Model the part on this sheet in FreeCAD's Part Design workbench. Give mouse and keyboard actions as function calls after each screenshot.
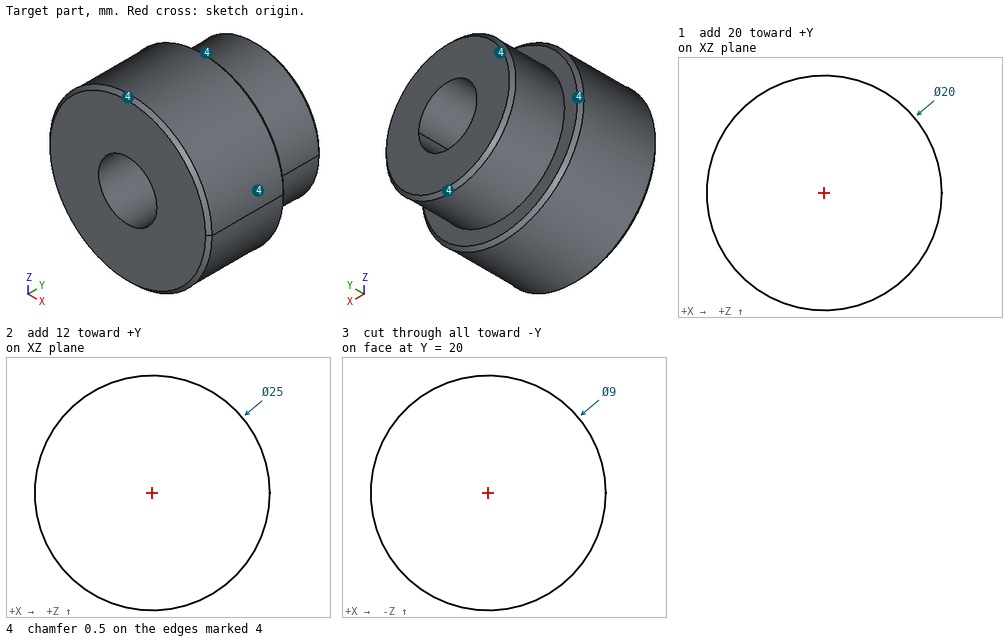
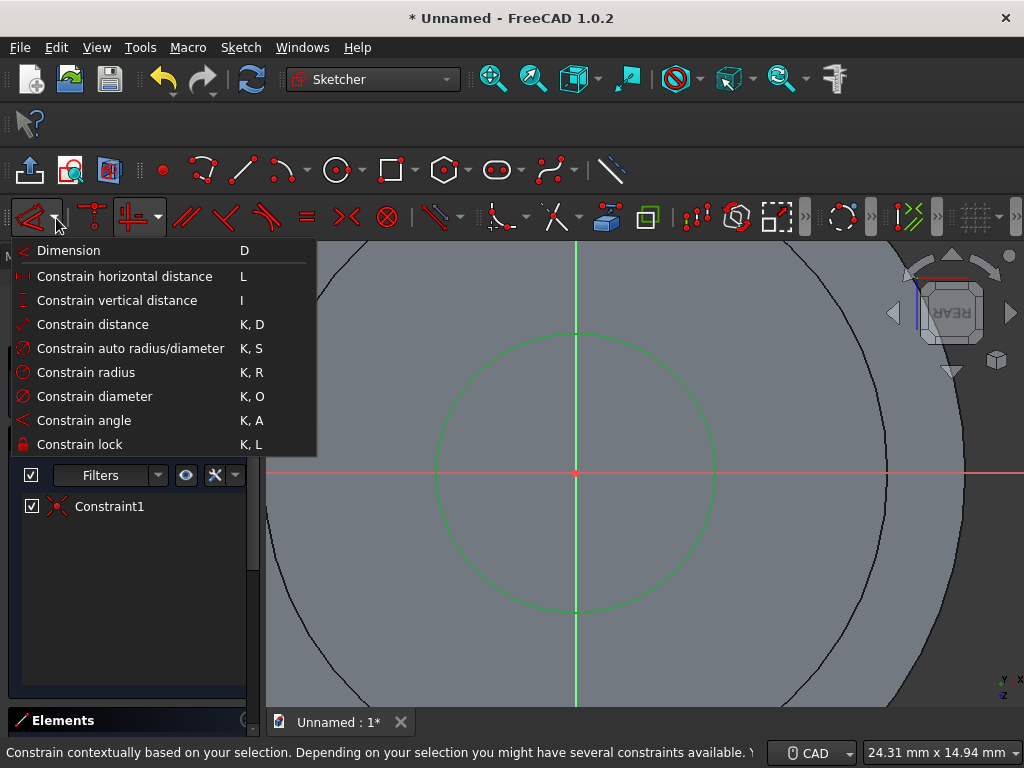
click(164, 396)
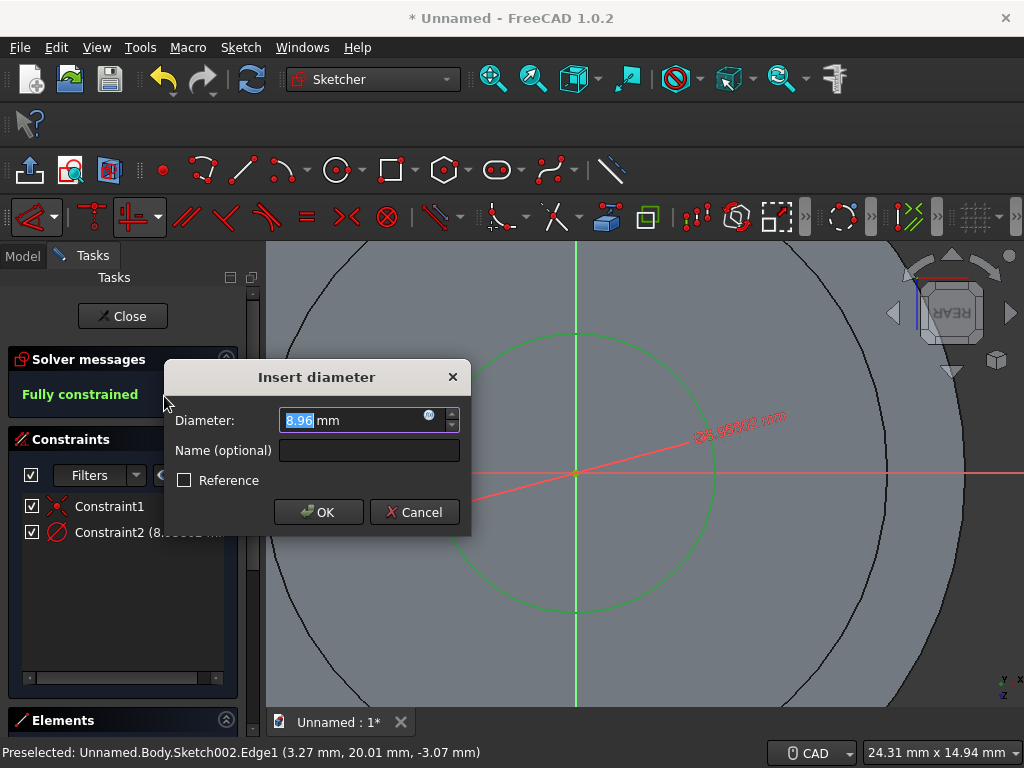
text(9)
key(Return)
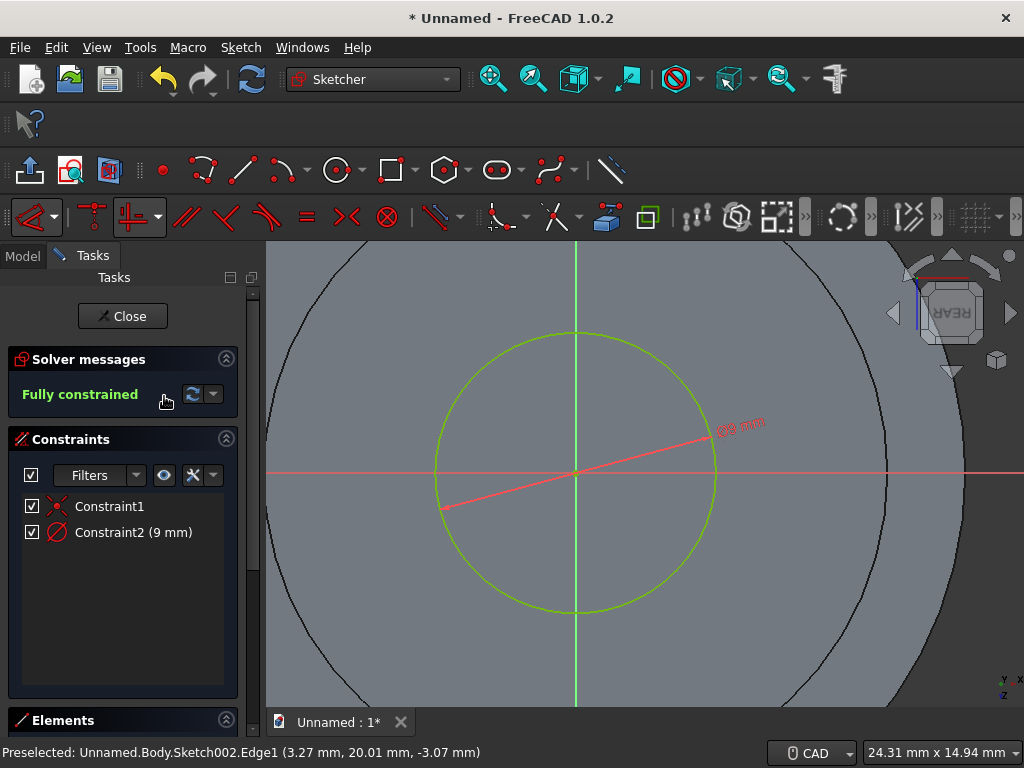
click(123, 316)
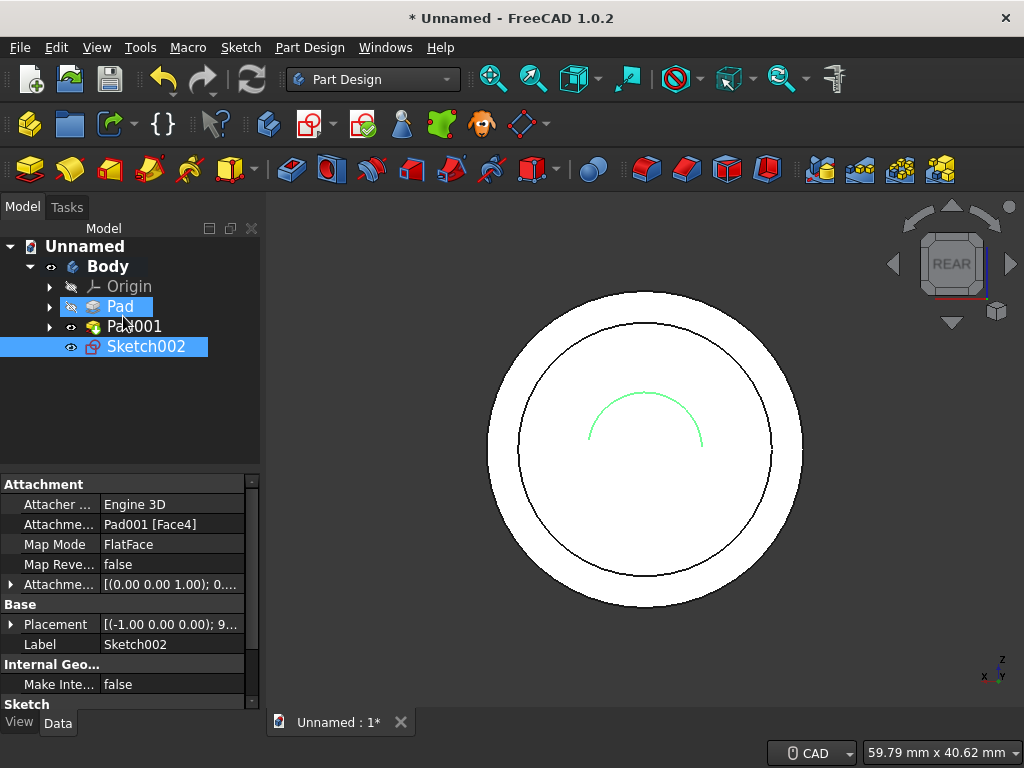
click(292, 170)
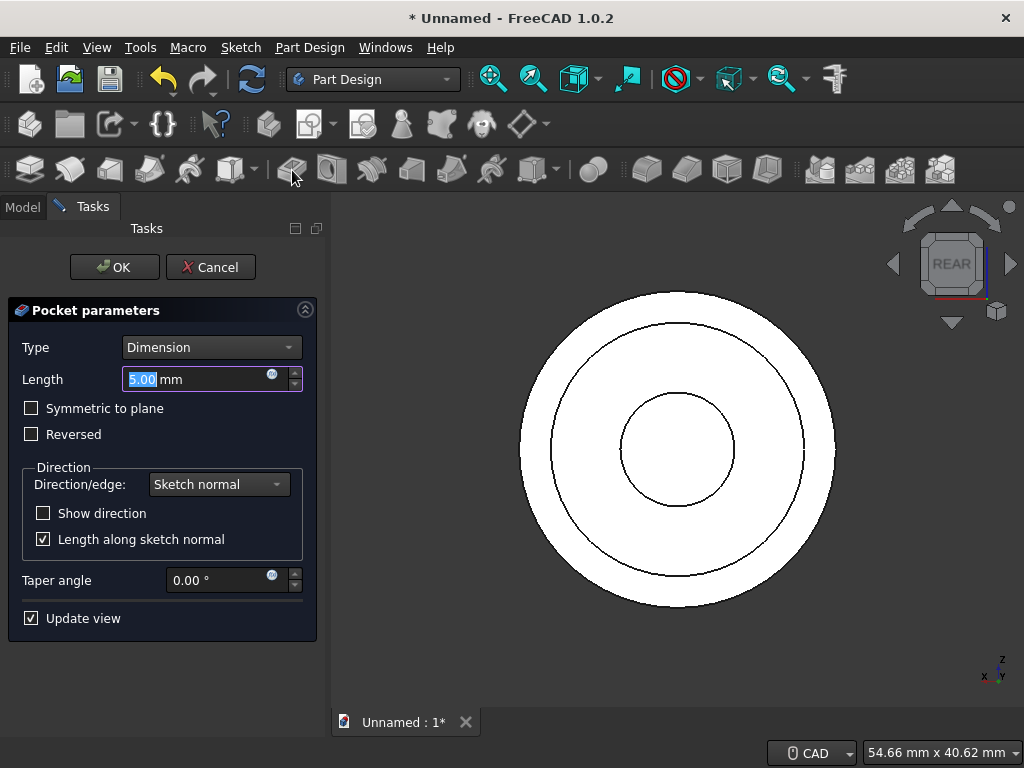
click(212, 348)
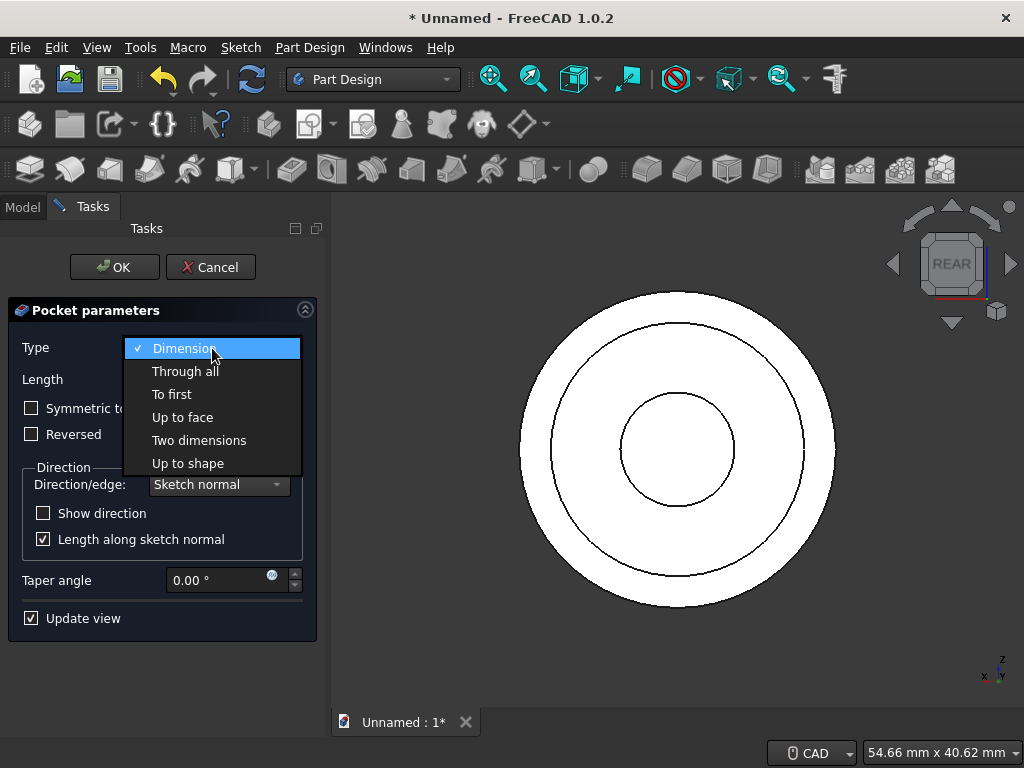
click(212, 372)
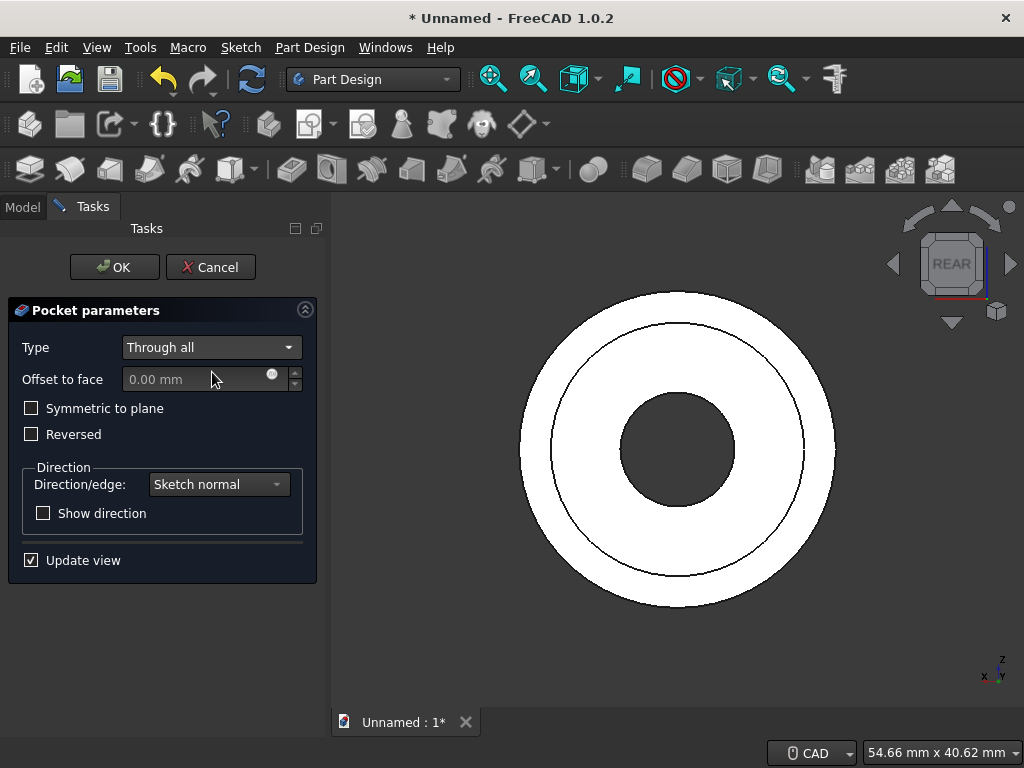
click(115, 267)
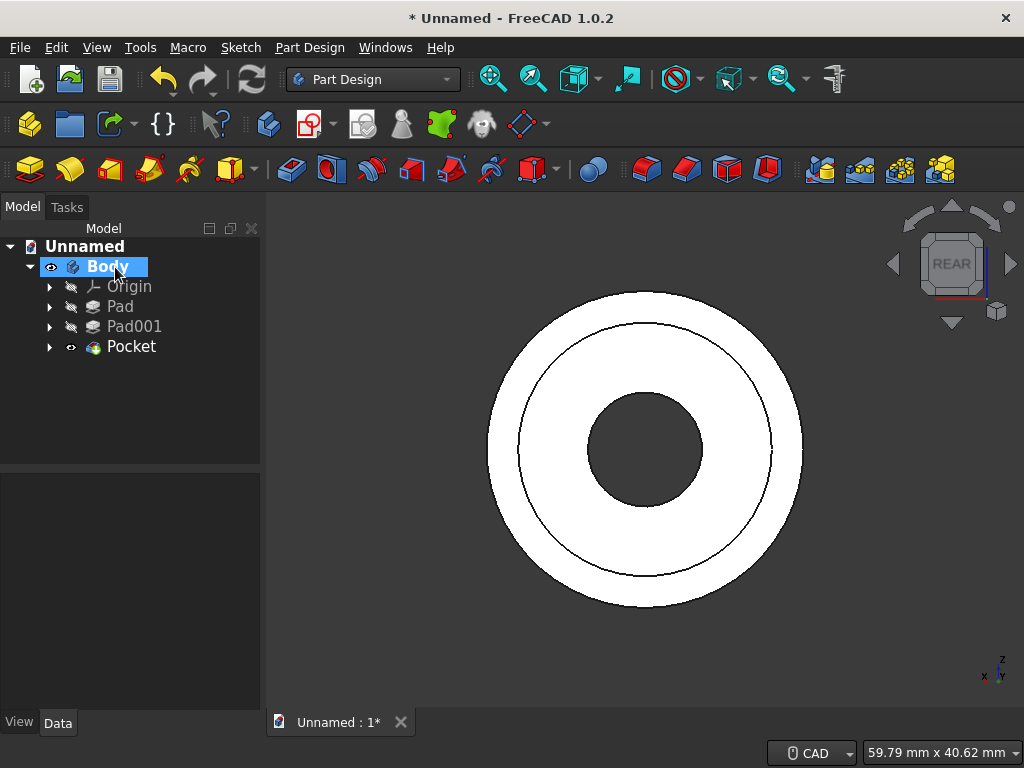
click(772, 449)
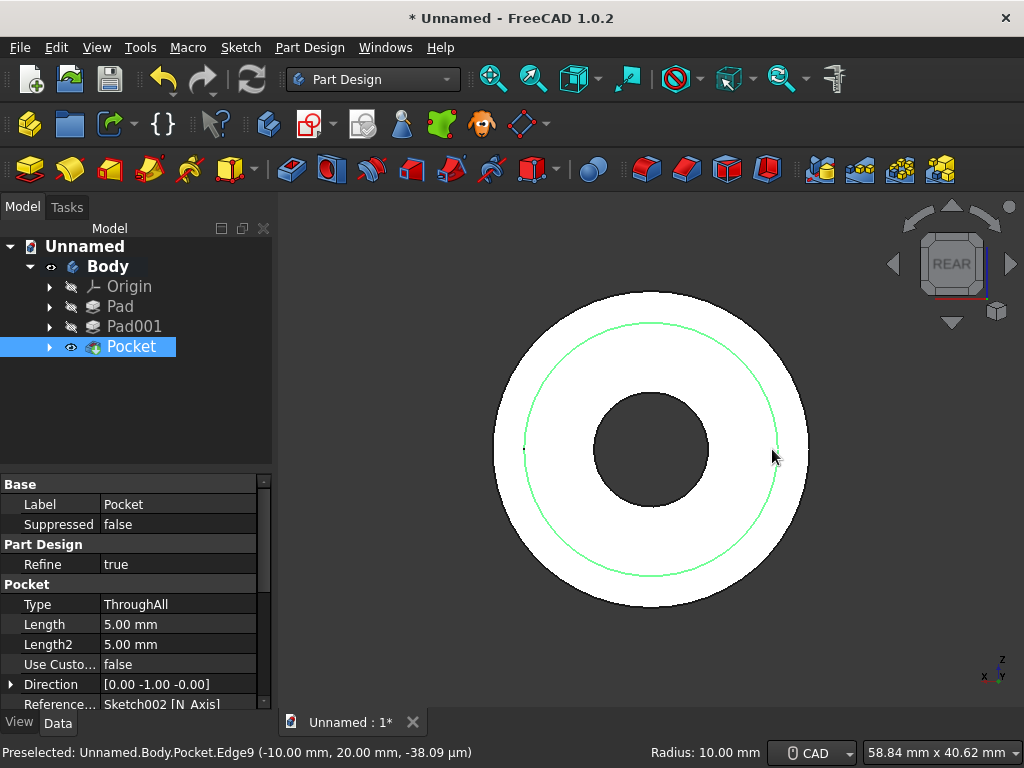
click(809, 449, ctrl)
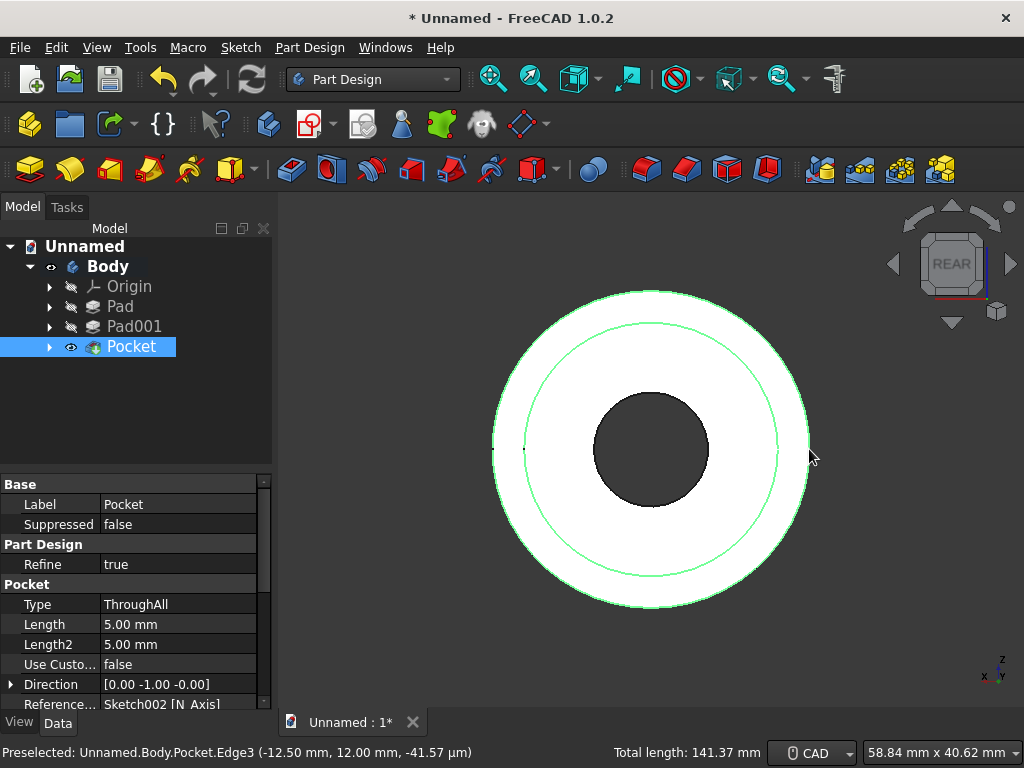
key(0)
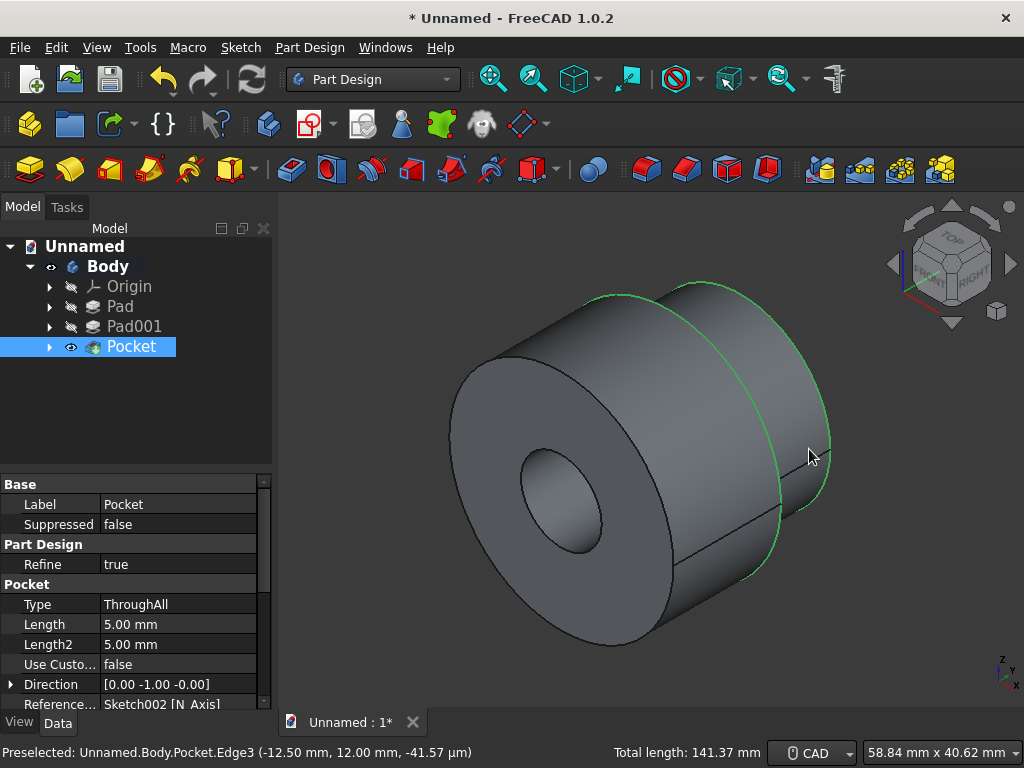
click(527, 357, ctrl)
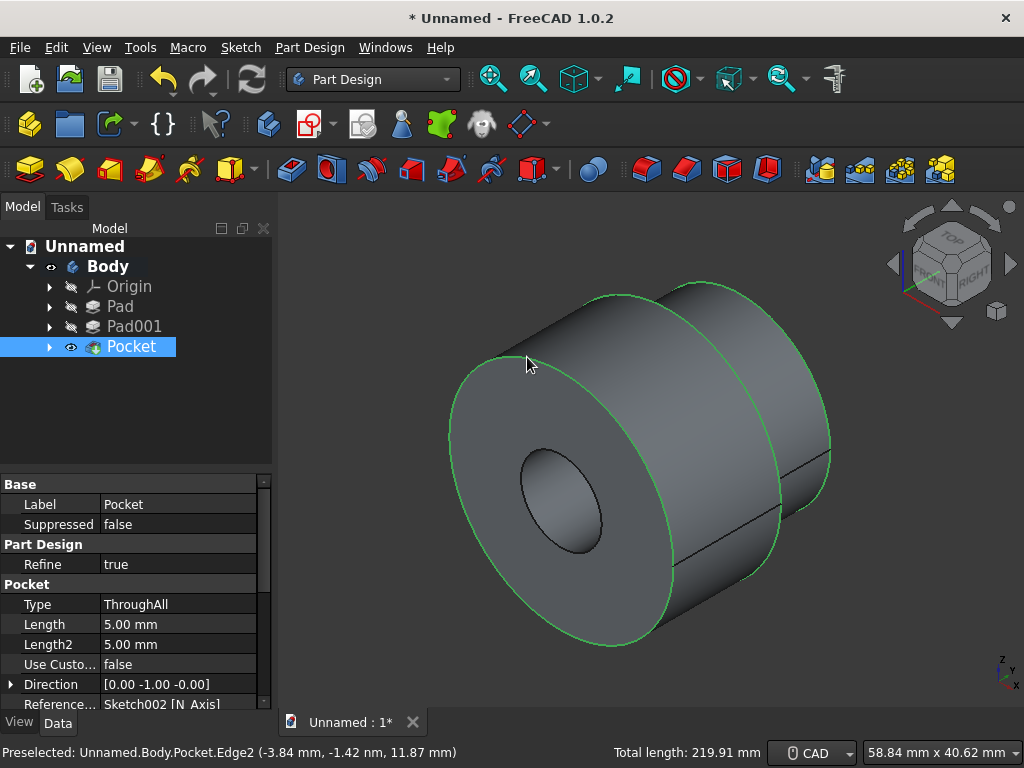
click(688, 170)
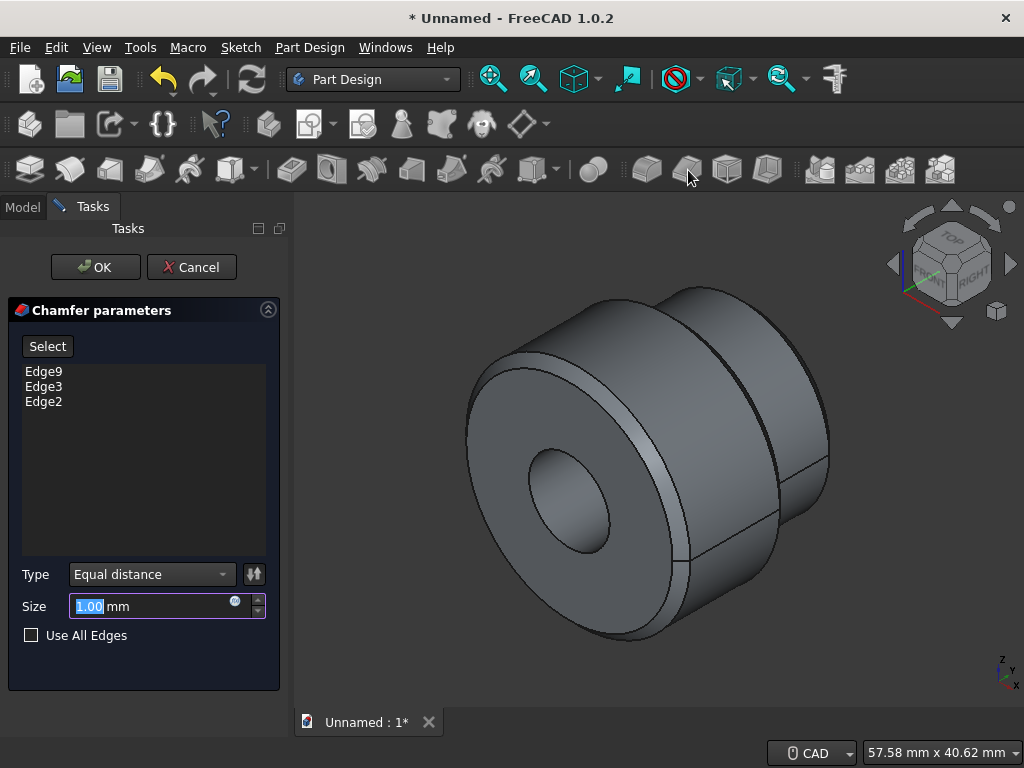
text(0.5)
key(Tab)